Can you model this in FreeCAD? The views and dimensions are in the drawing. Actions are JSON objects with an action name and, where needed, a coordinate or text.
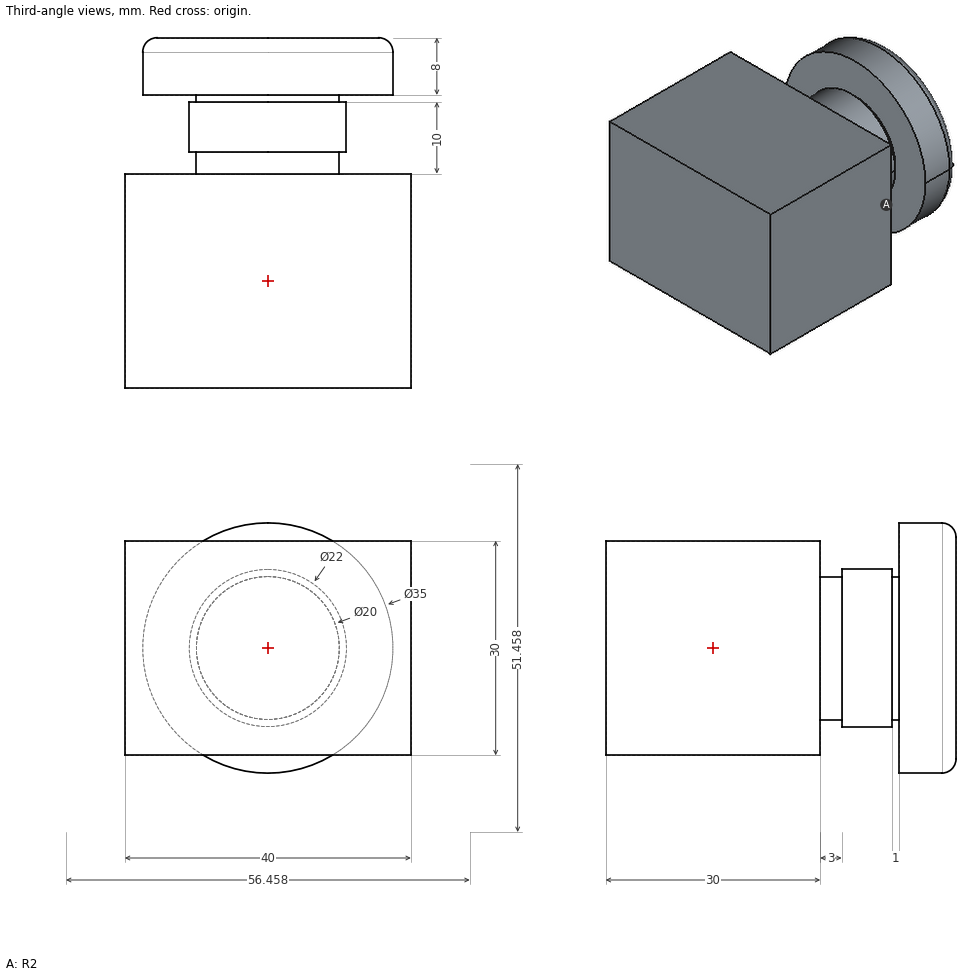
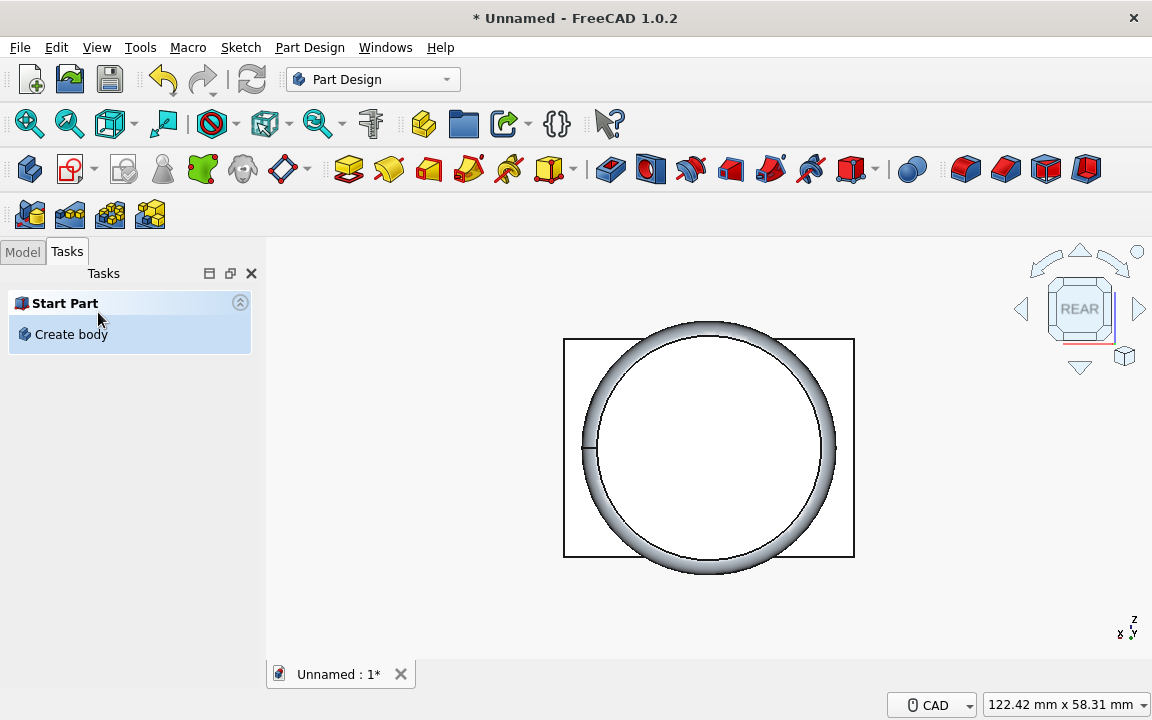
{"action": "left_click", "coordinate": [23, 251]}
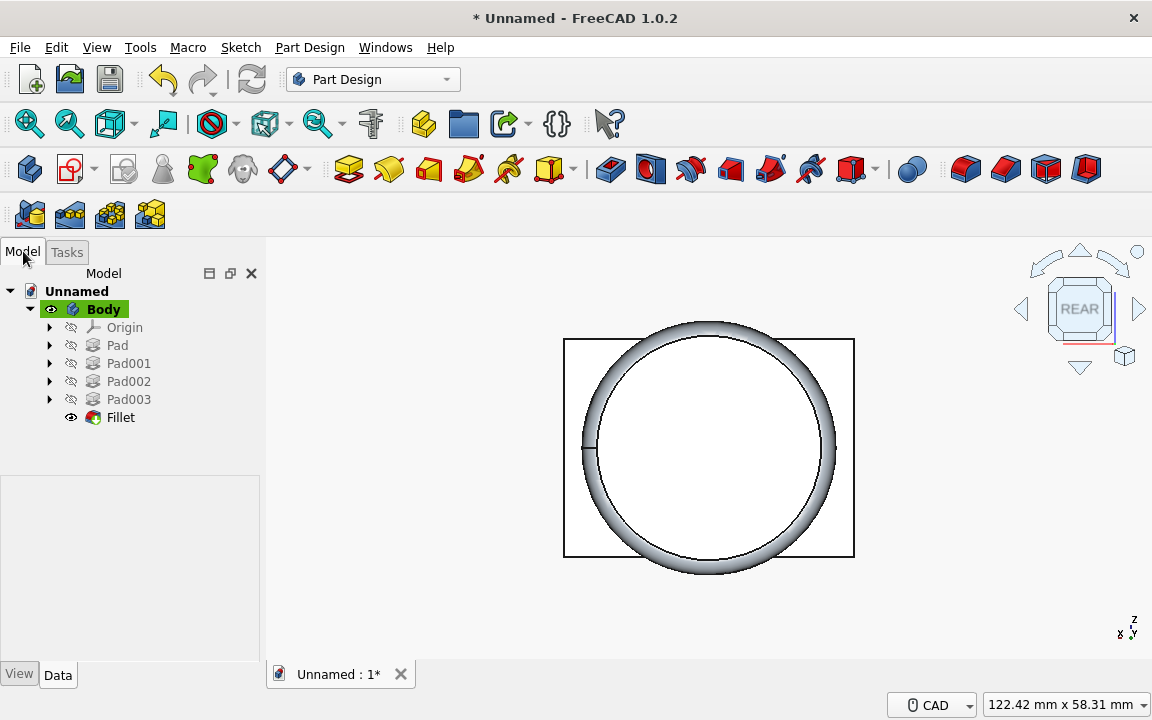
{"action": "left_click", "coordinate": [50, 327]}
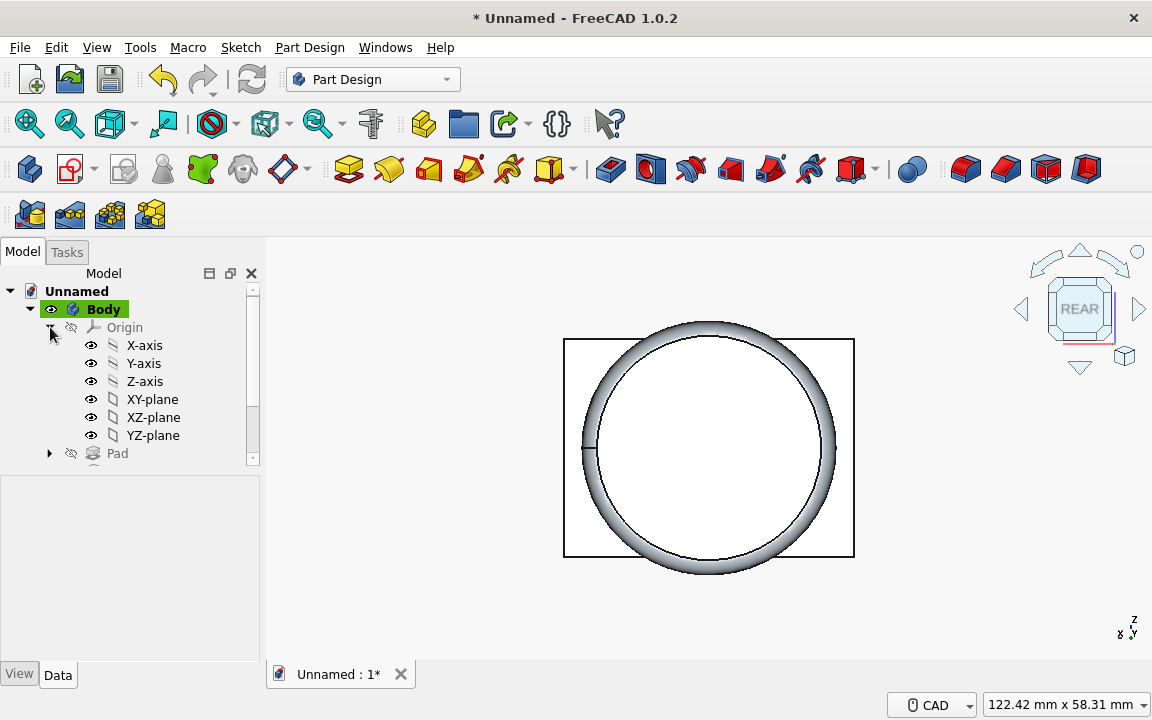
{"action": "left_click", "coordinate": [136, 417]}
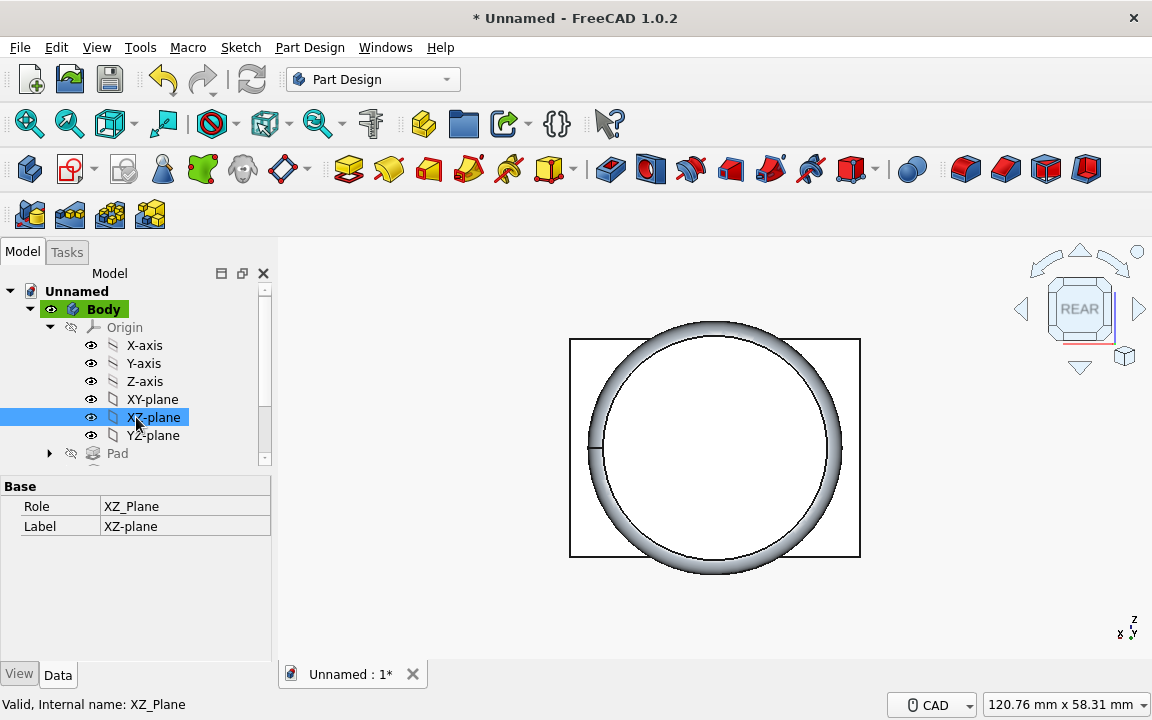
{"action": "left_click", "coordinate": [284, 170]}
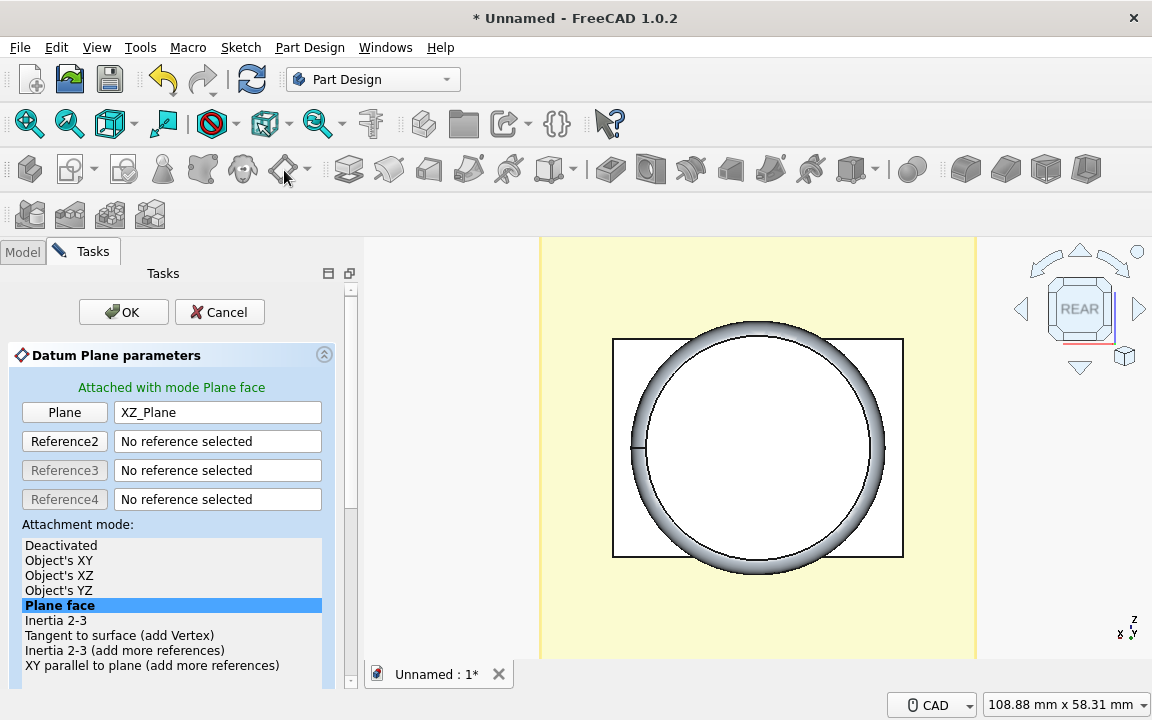
{"action": "scroll", "coordinate": [351, 486], "scroll_direction": "down", "scroll_amount": 4}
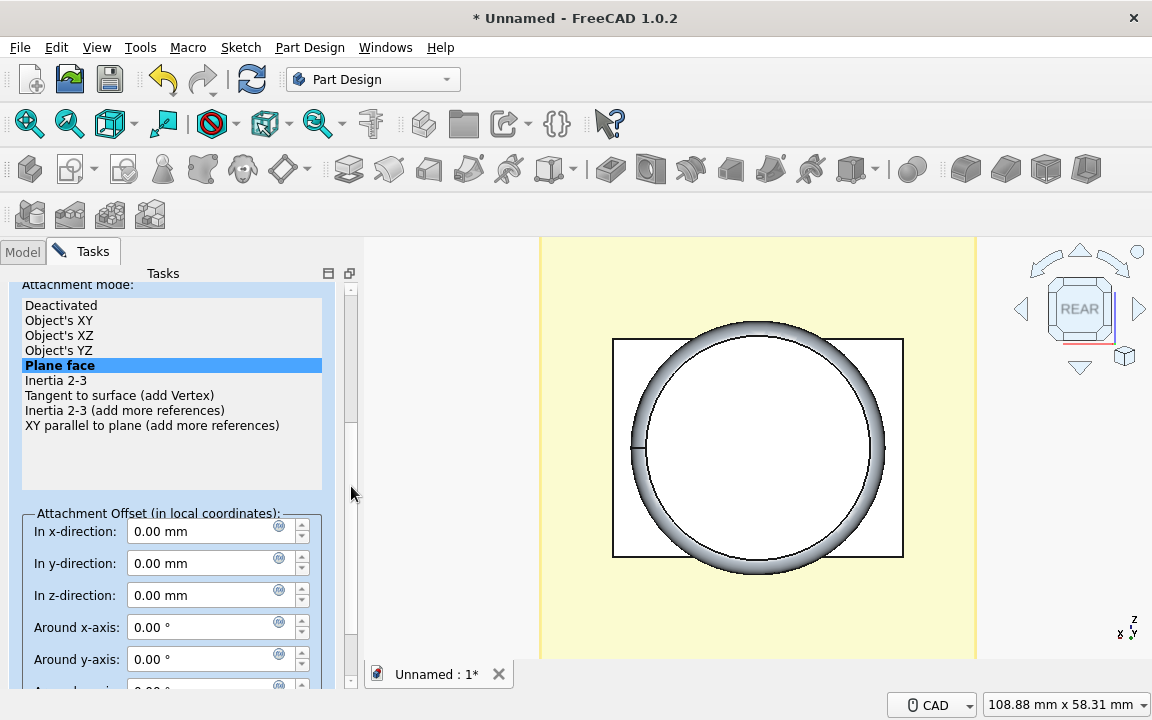
{"action": "triple_click", "coordinate": [210, 595]}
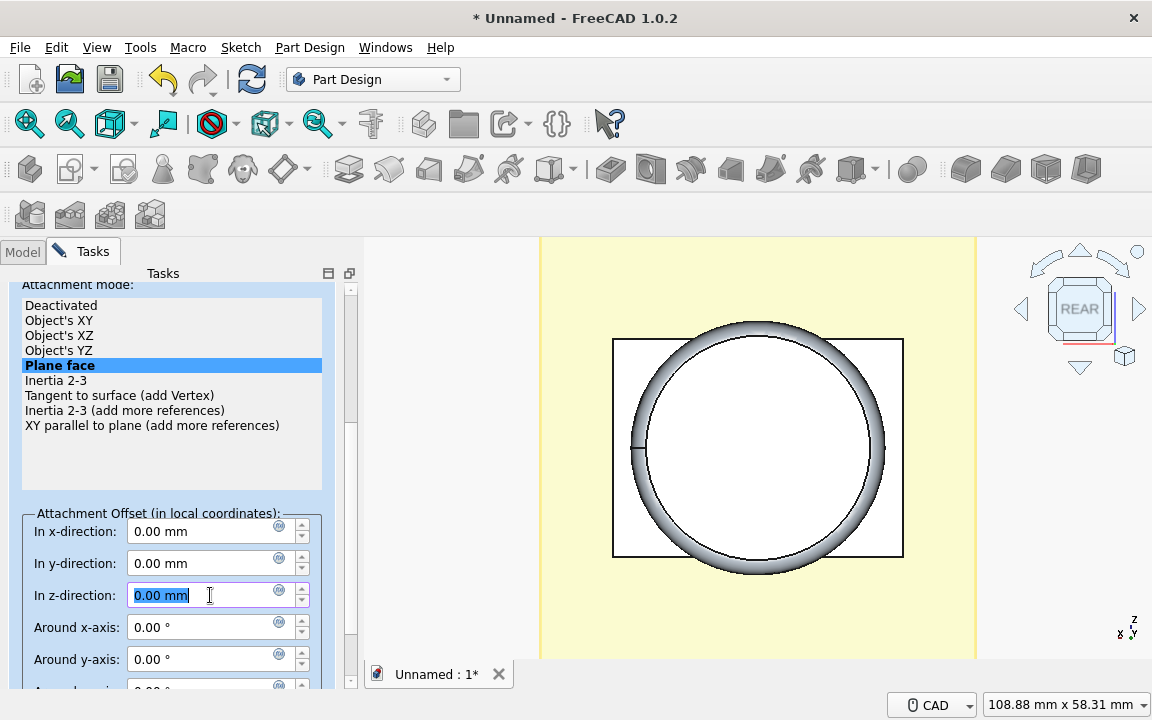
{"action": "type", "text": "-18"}
{"action": "key", "text": "Tab"}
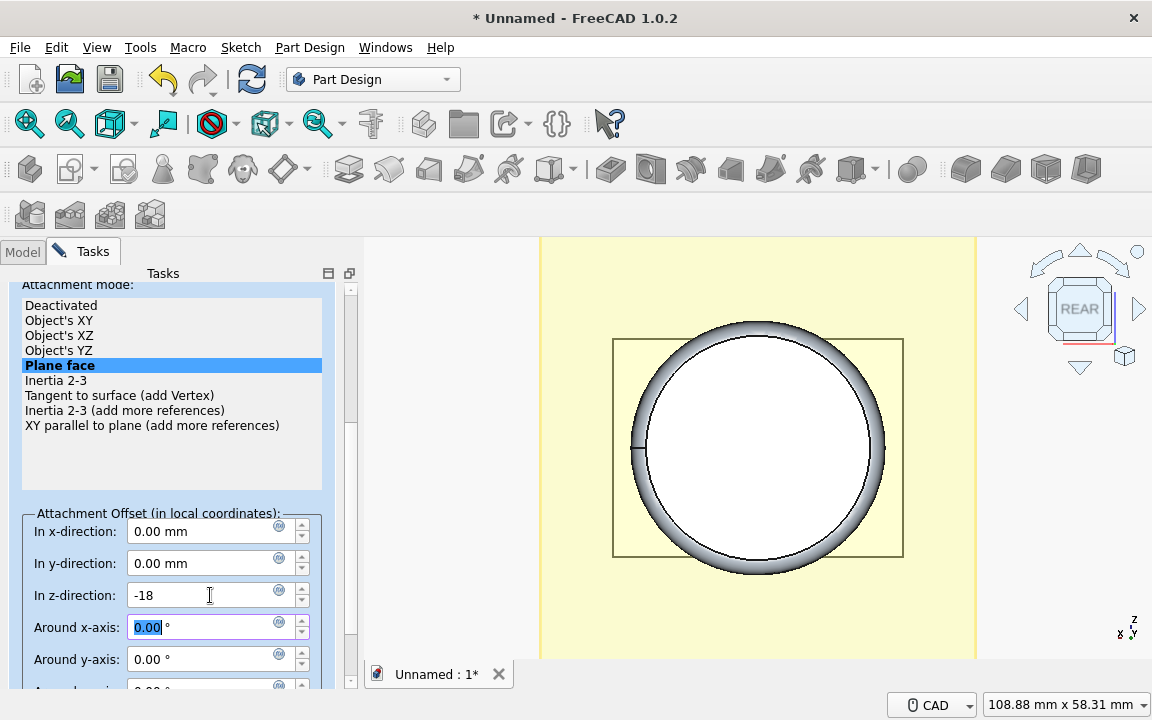
{"action": "scroll", "coordinate": [351, 486], "scroll_direction": "up", "scroll_amount": 5}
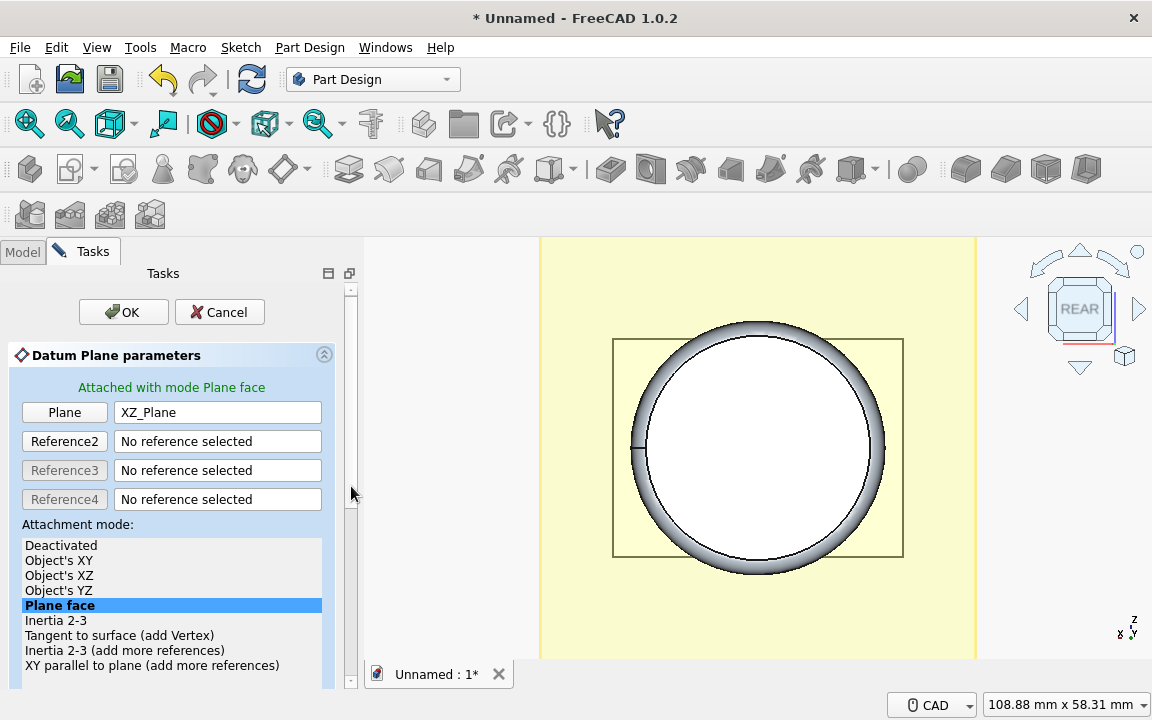
{"action": "left_click", "coordinate": [124, 312]}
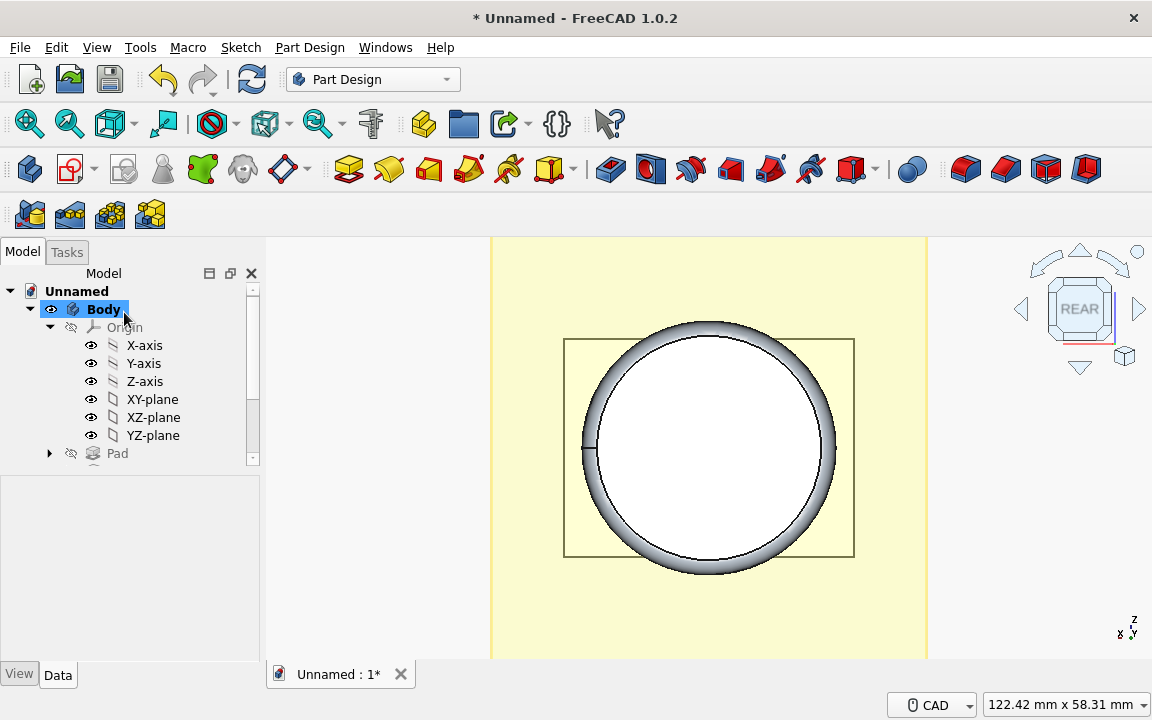
{"action": "scroll", "coordinate": [100, 377], "scroll_direction": "down", "scroll_amount": 3}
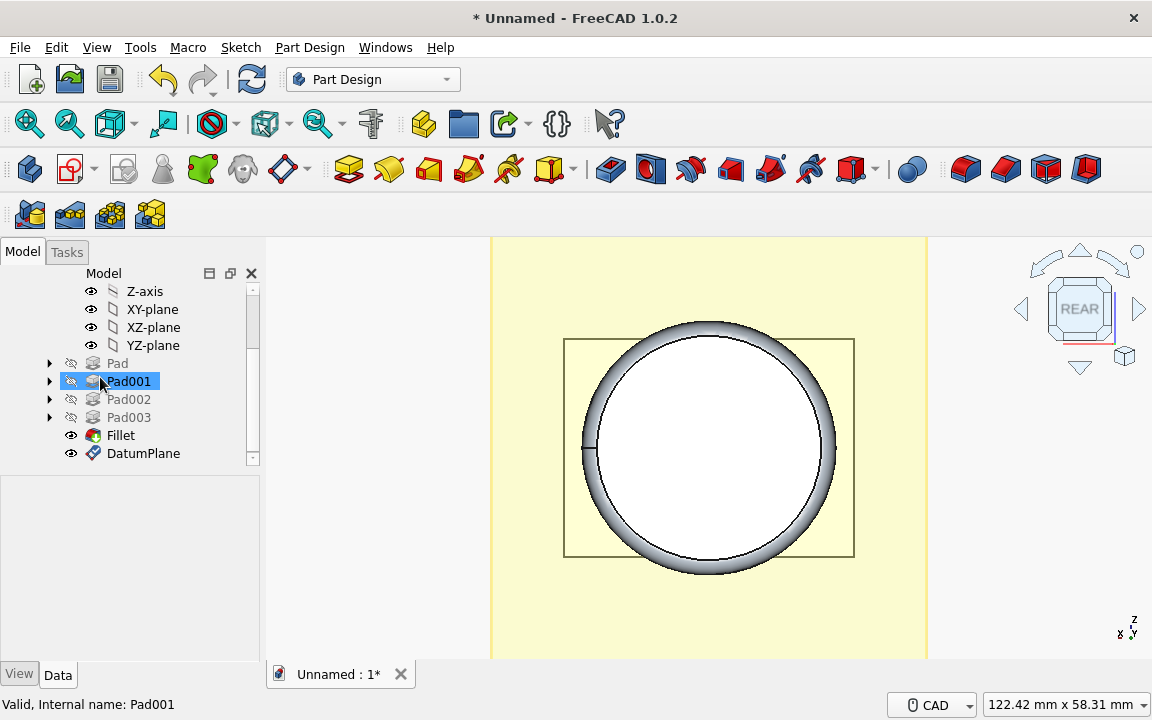
{"action": "left_click", "coordinate": [116, 453]}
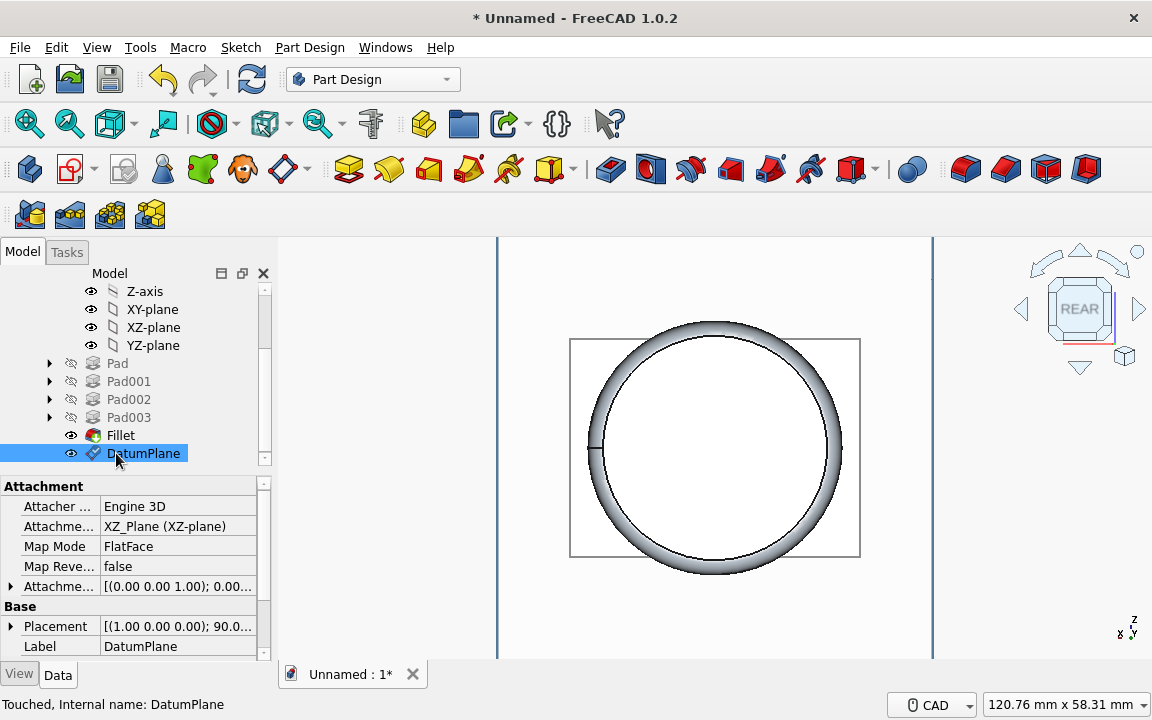
{"action": "left_click", "coordinate": [70, 170]}